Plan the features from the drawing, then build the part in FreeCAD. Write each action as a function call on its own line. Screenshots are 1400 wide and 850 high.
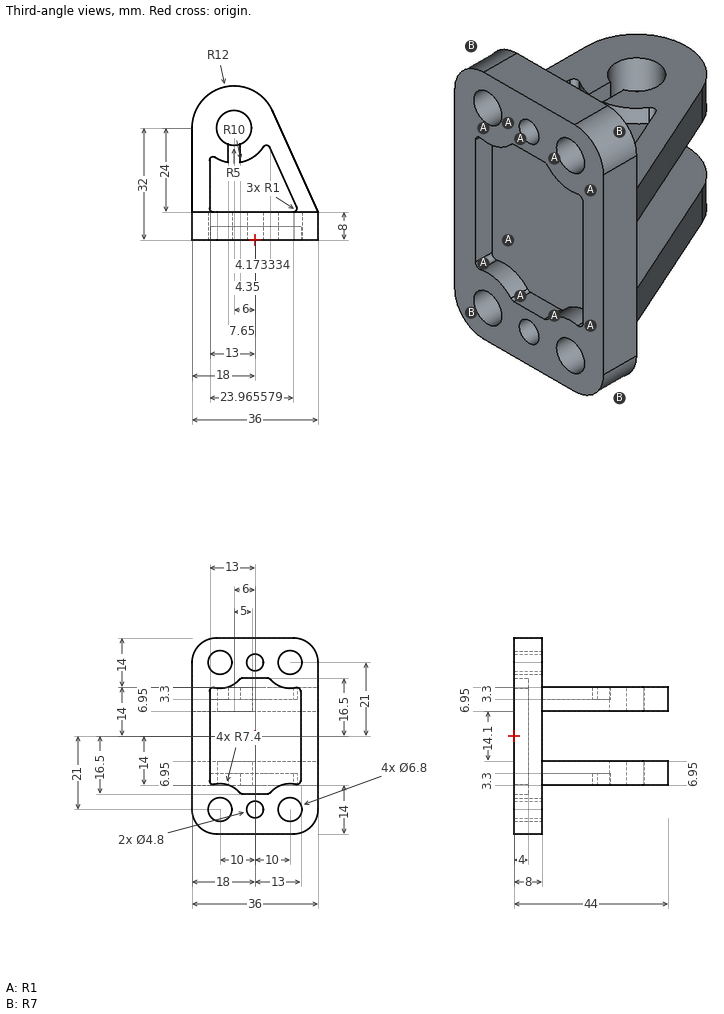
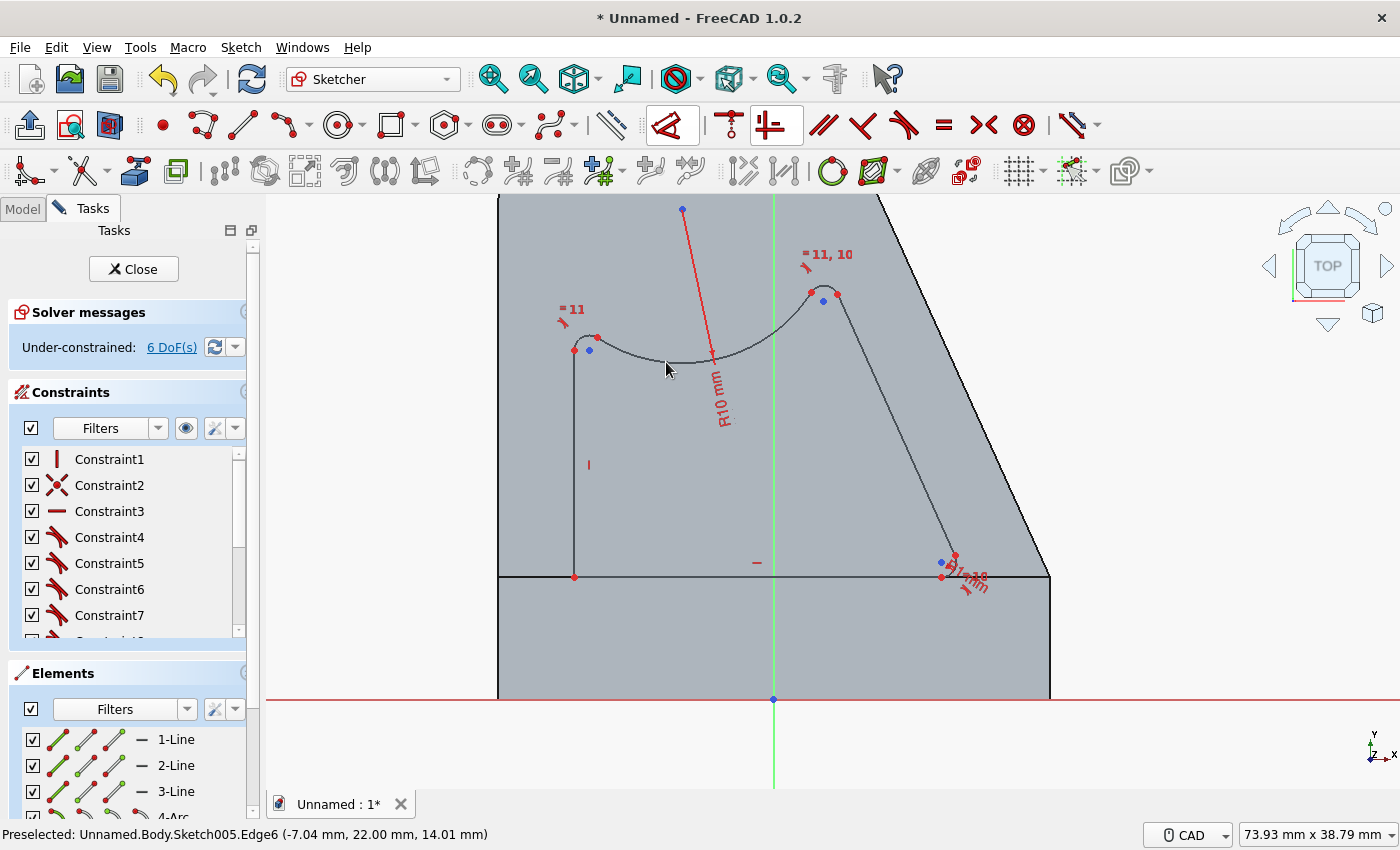
click(574, 577)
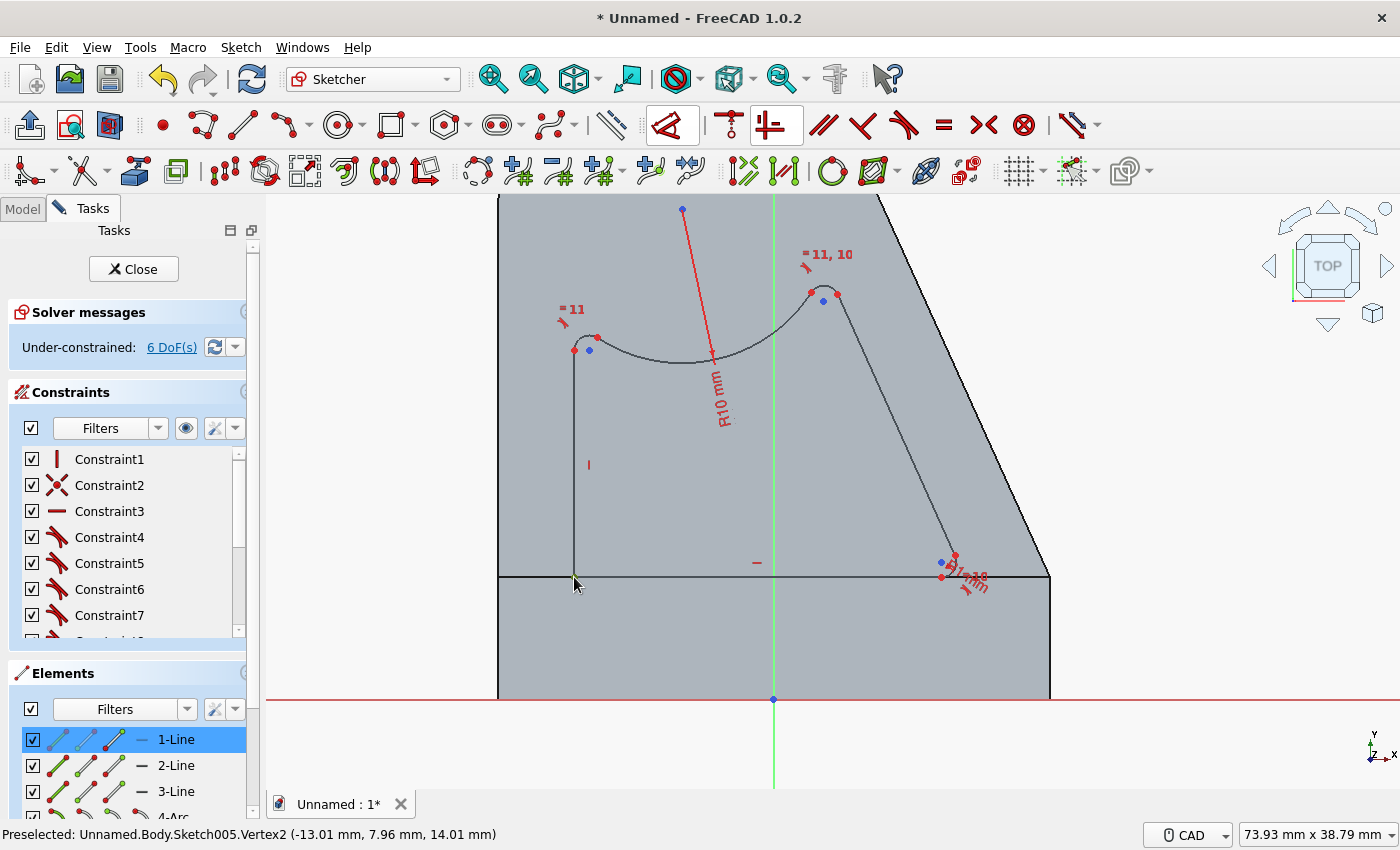
key(i)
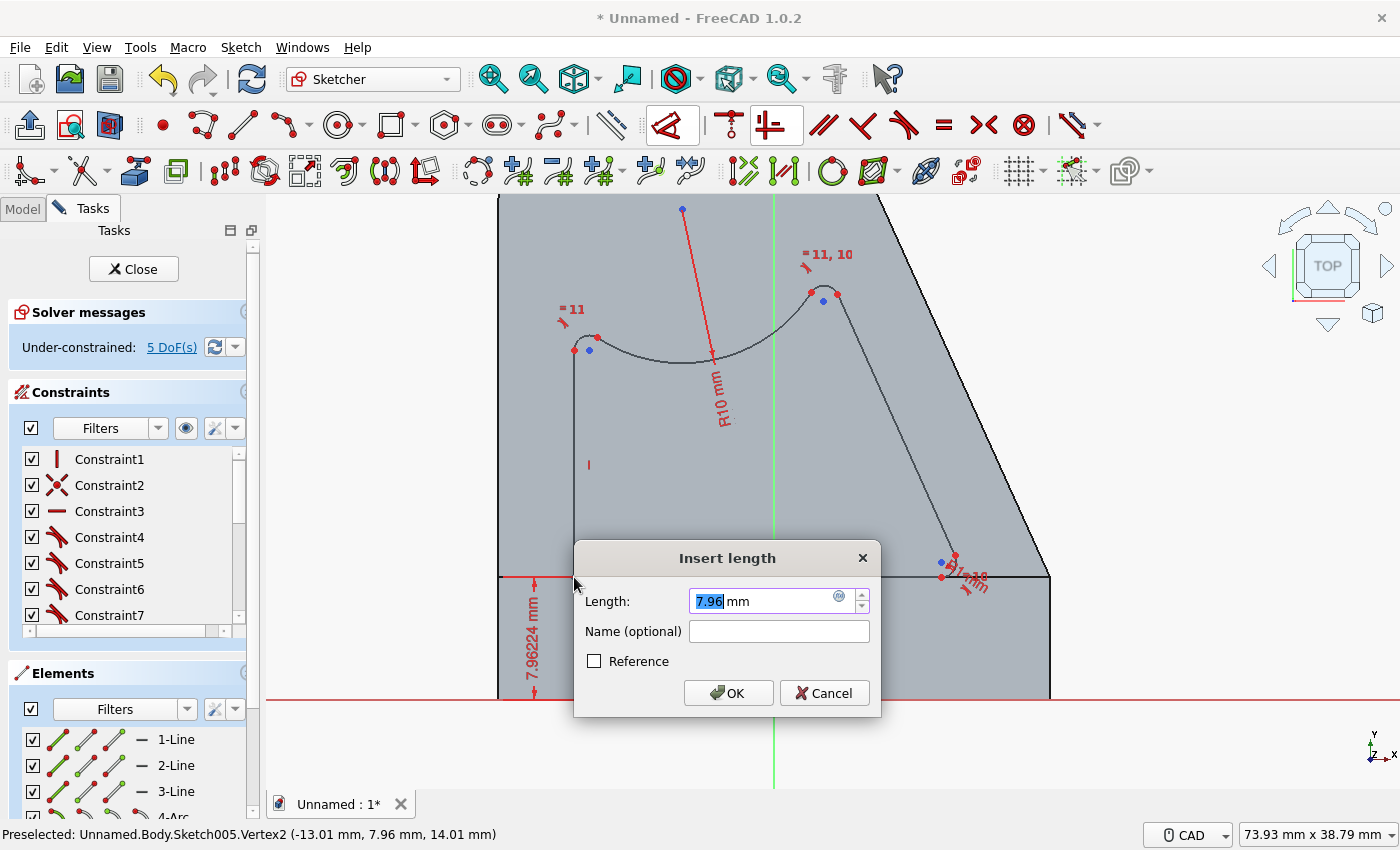
text(8)
key(Return)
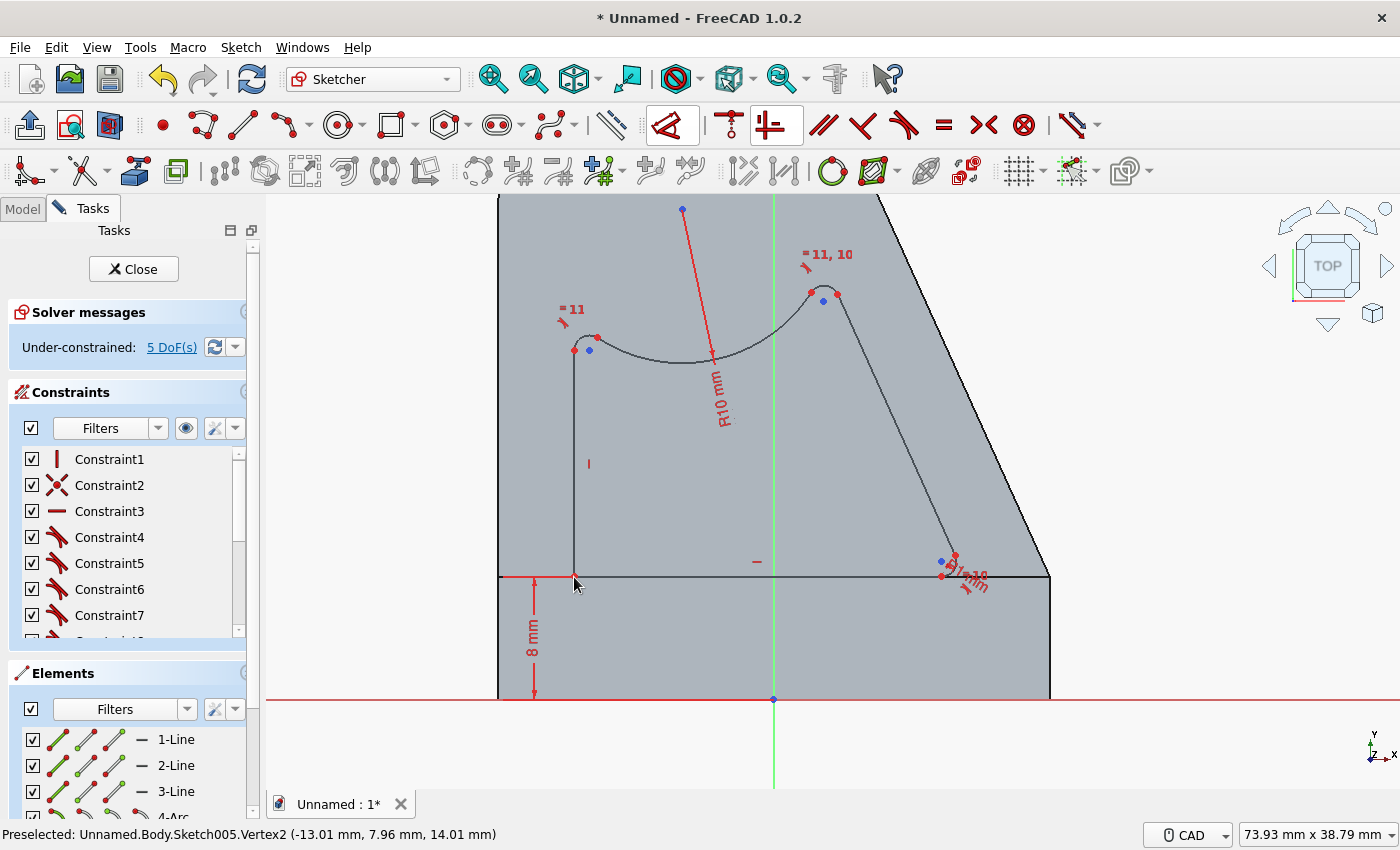
scroll(762, 658, down, 1)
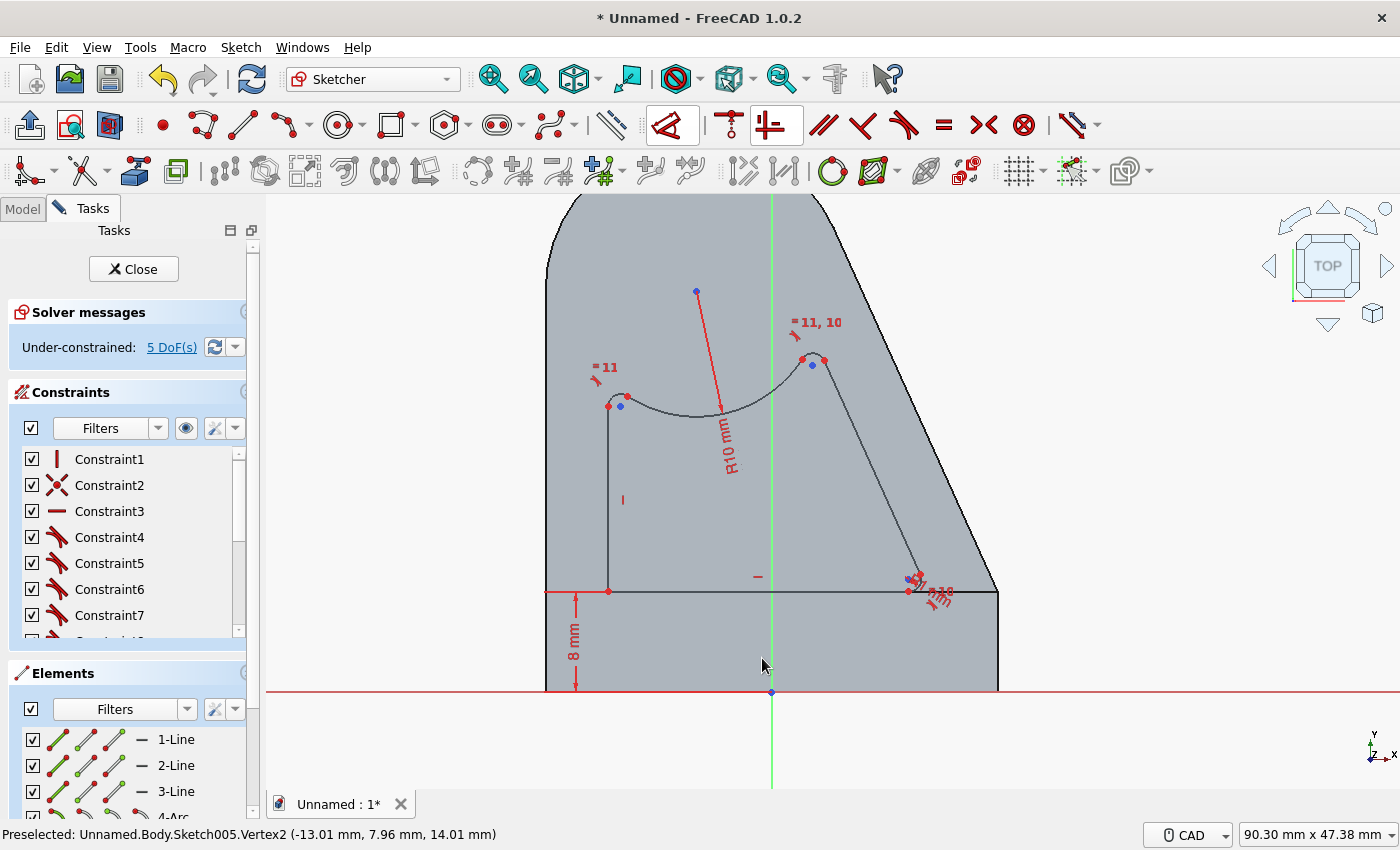
click(697, 291)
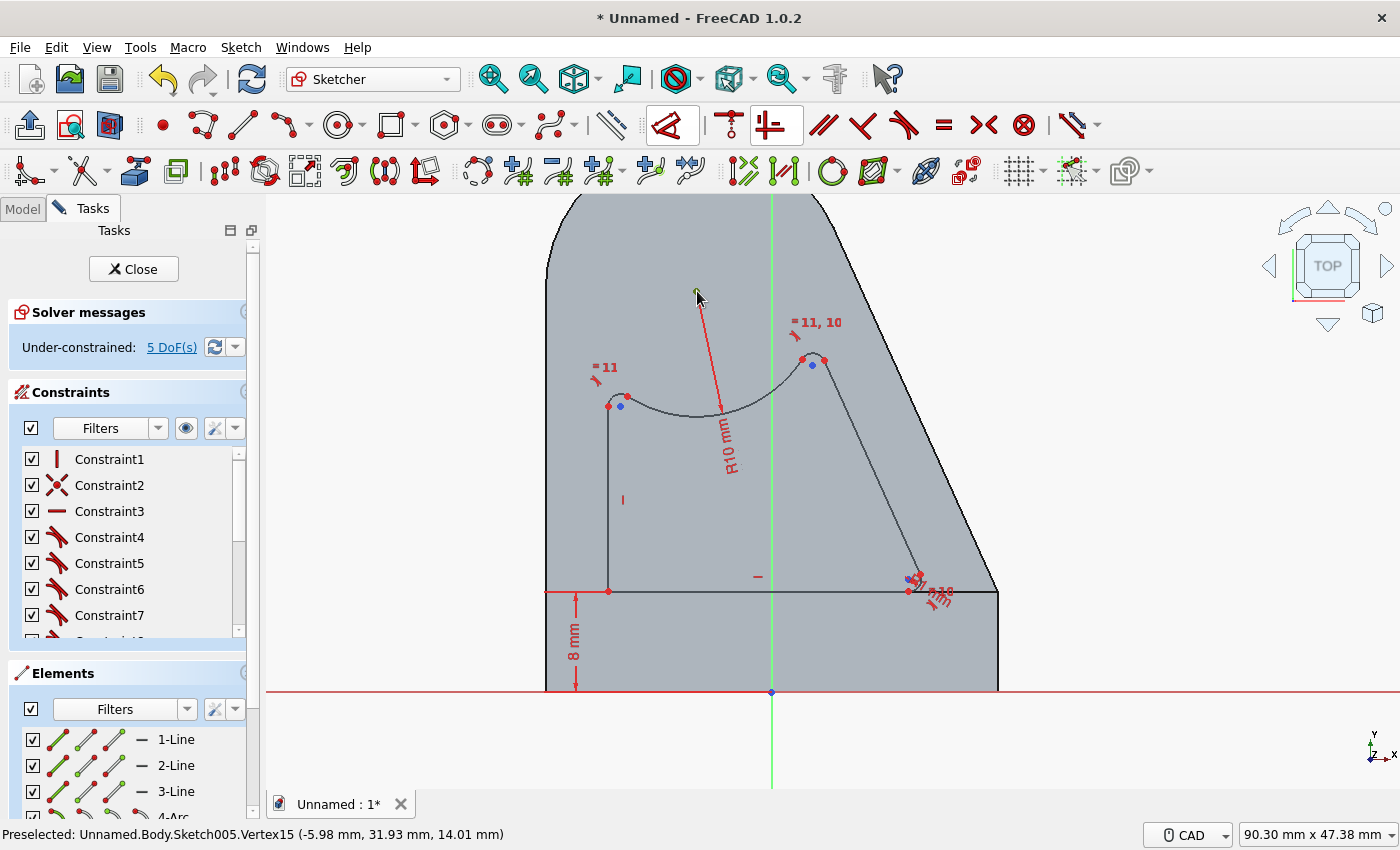
click(694, 126)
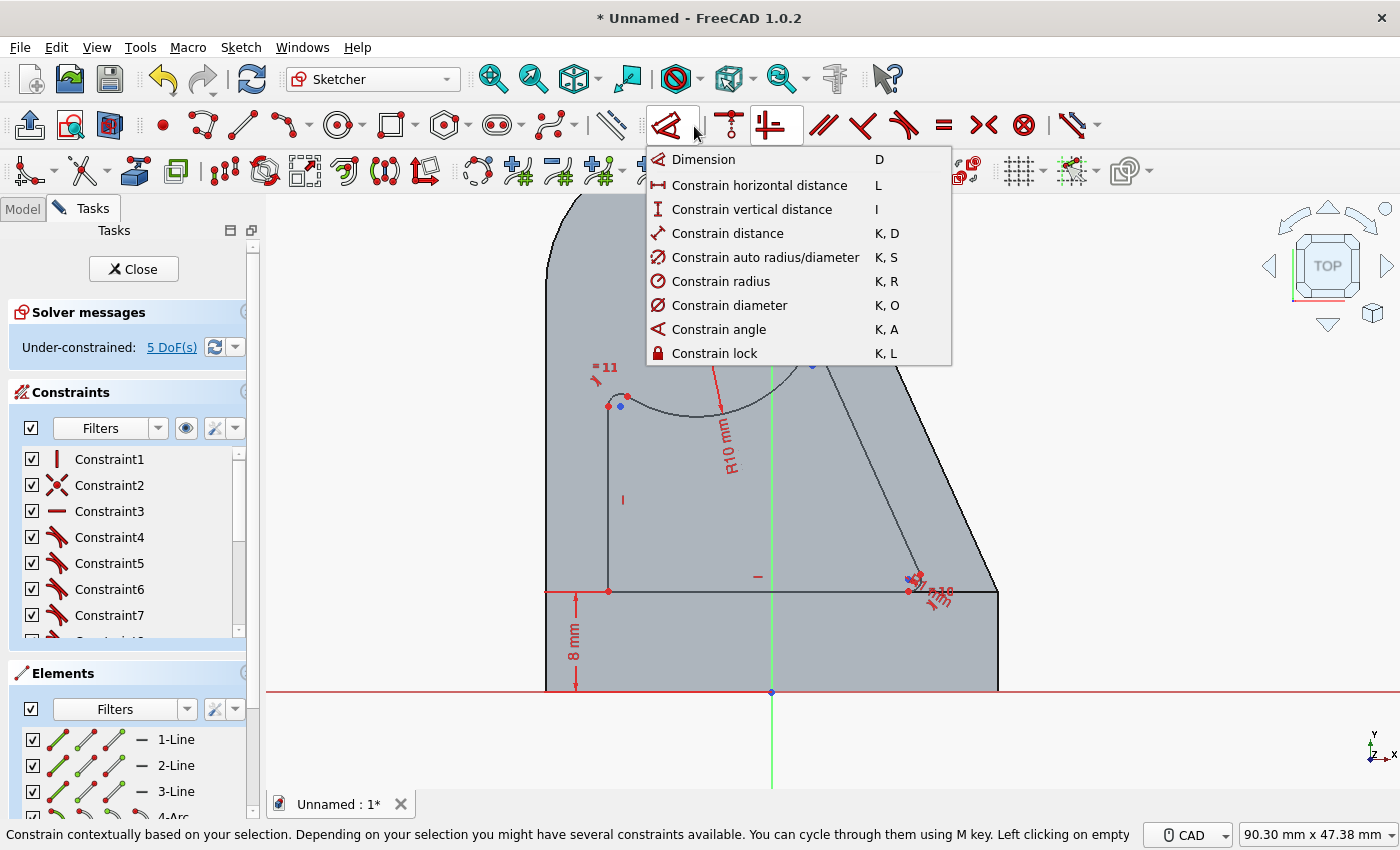
click(799, 185)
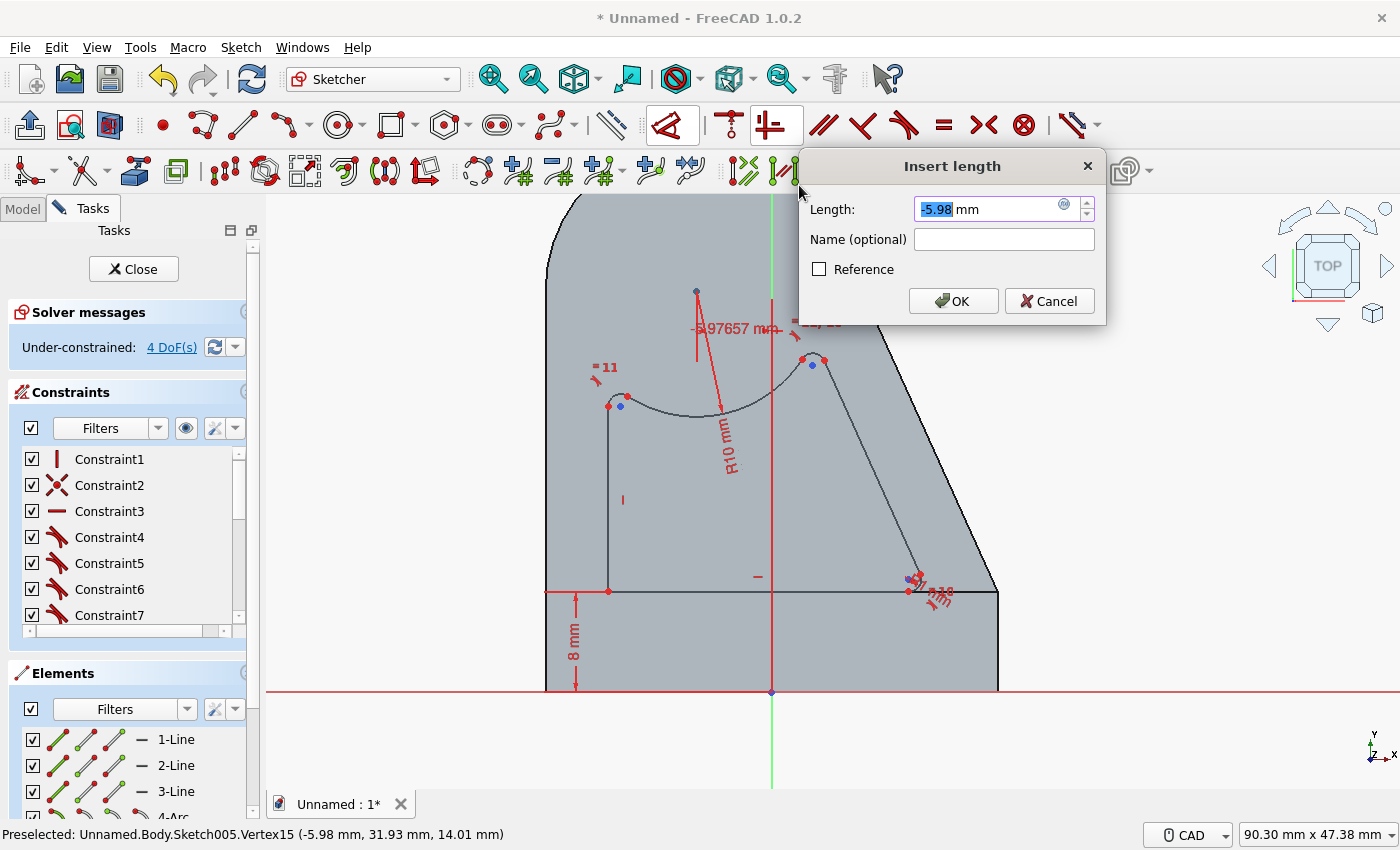
text(-6)
key(Return)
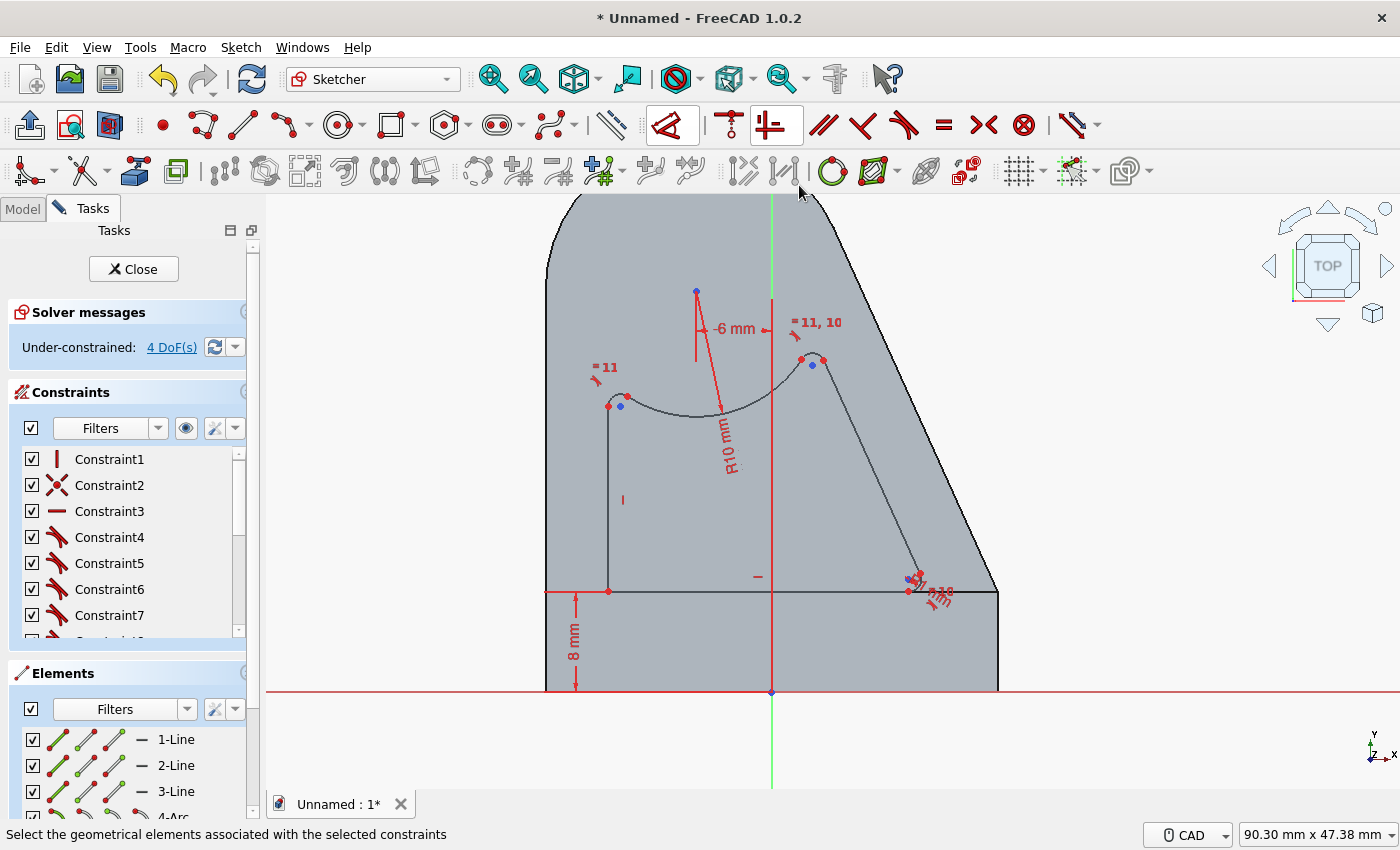
click(608, 407)